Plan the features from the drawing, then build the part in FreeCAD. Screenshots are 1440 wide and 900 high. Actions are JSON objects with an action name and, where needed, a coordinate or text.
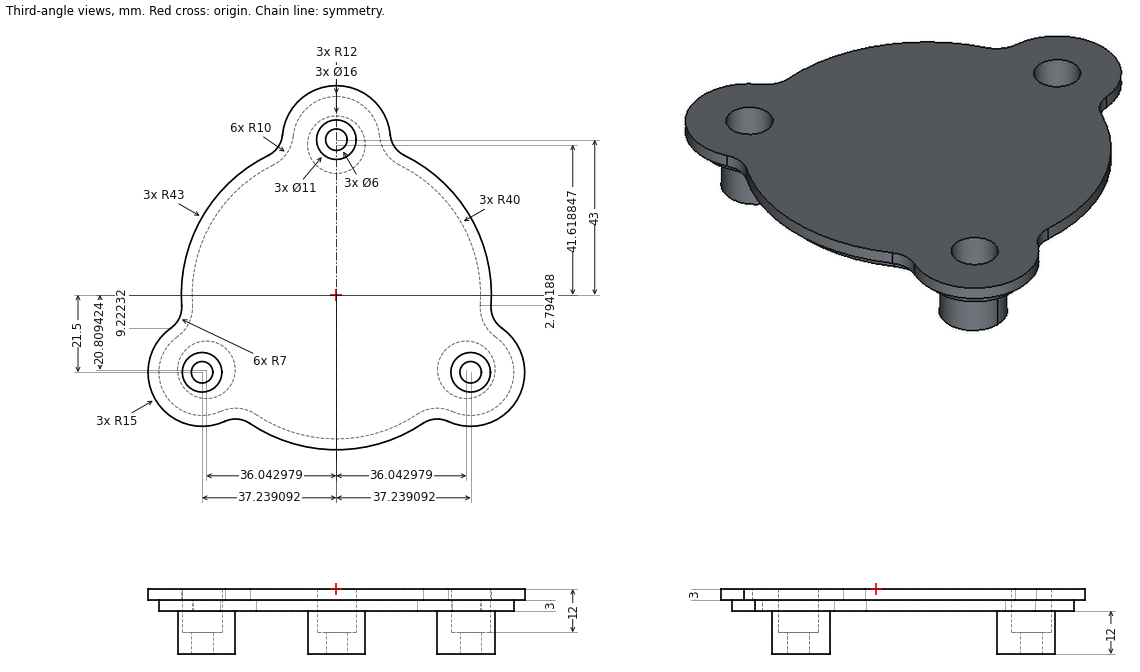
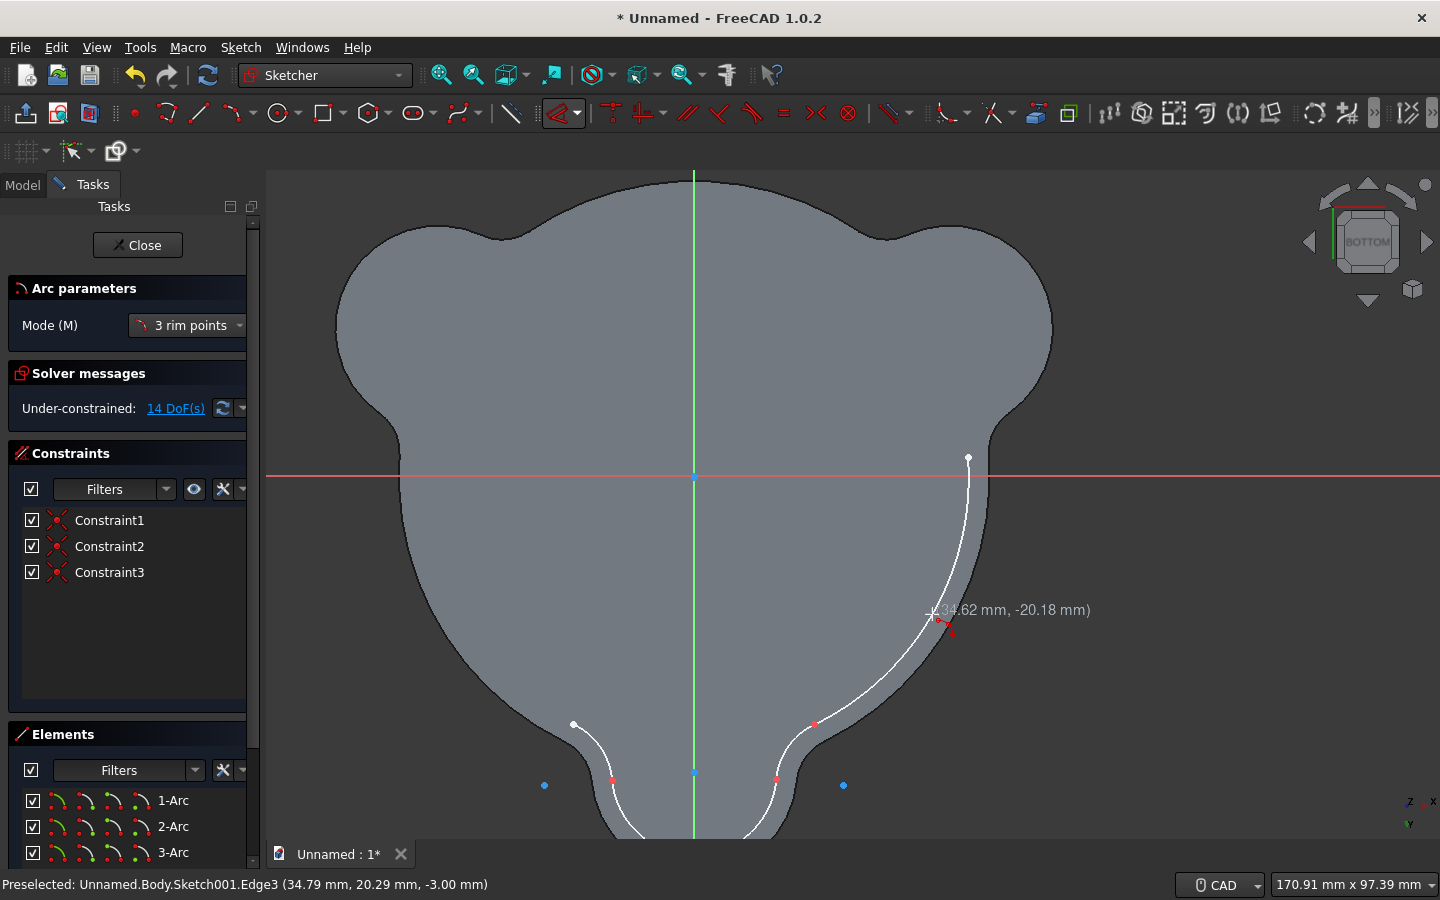
{"action": "left_click", "coordinate": [968, 458]}
{"action": "left_click", "coordinate": [997, 396]}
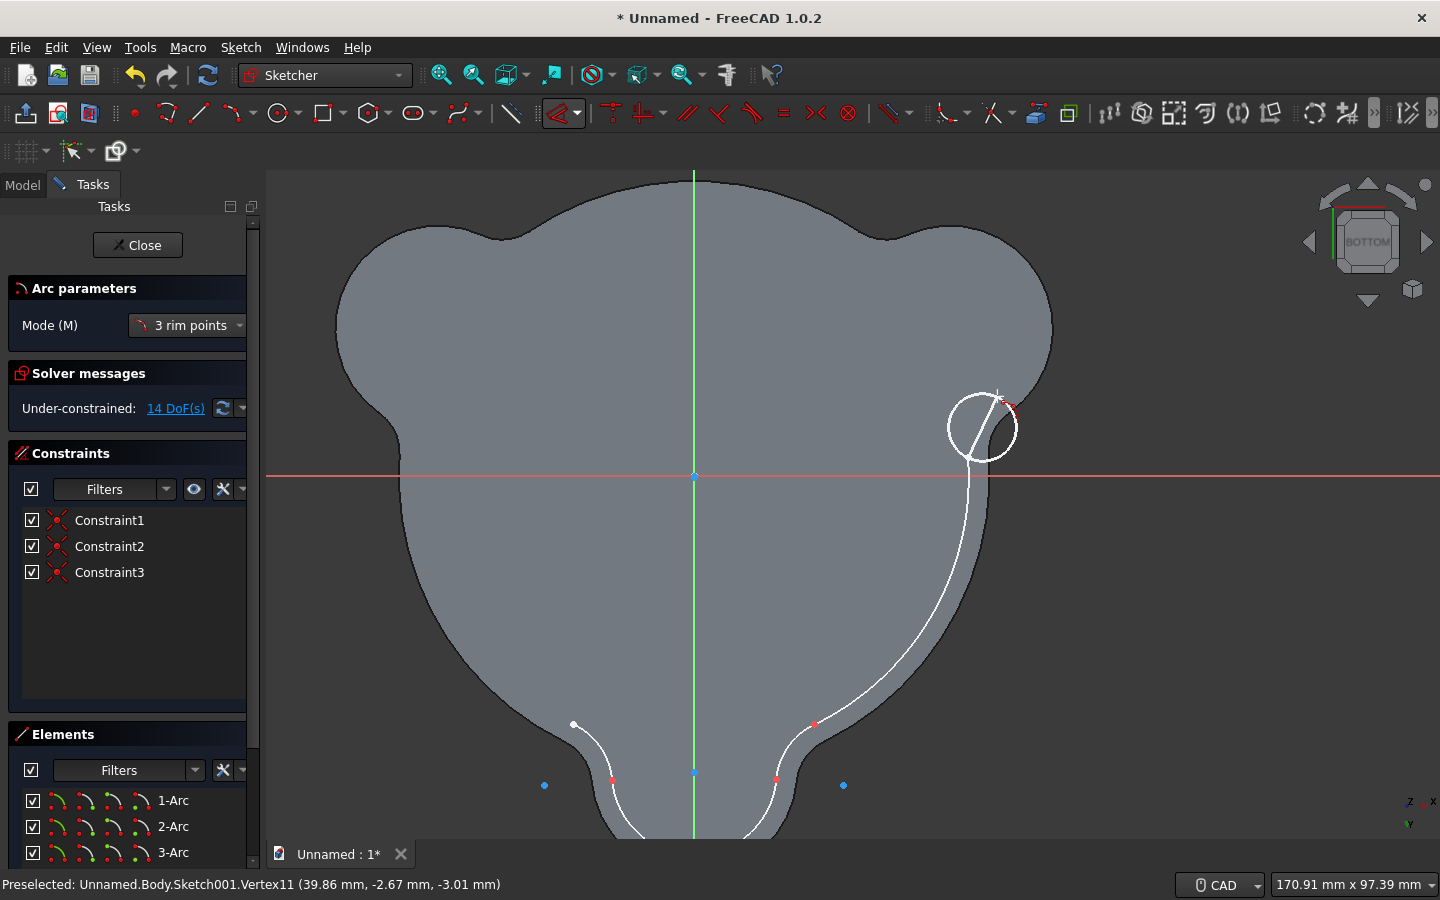
{"action": "scroll", "coordinate": [975, 423], "scroll_direction": "up", "scroll_amount": 3}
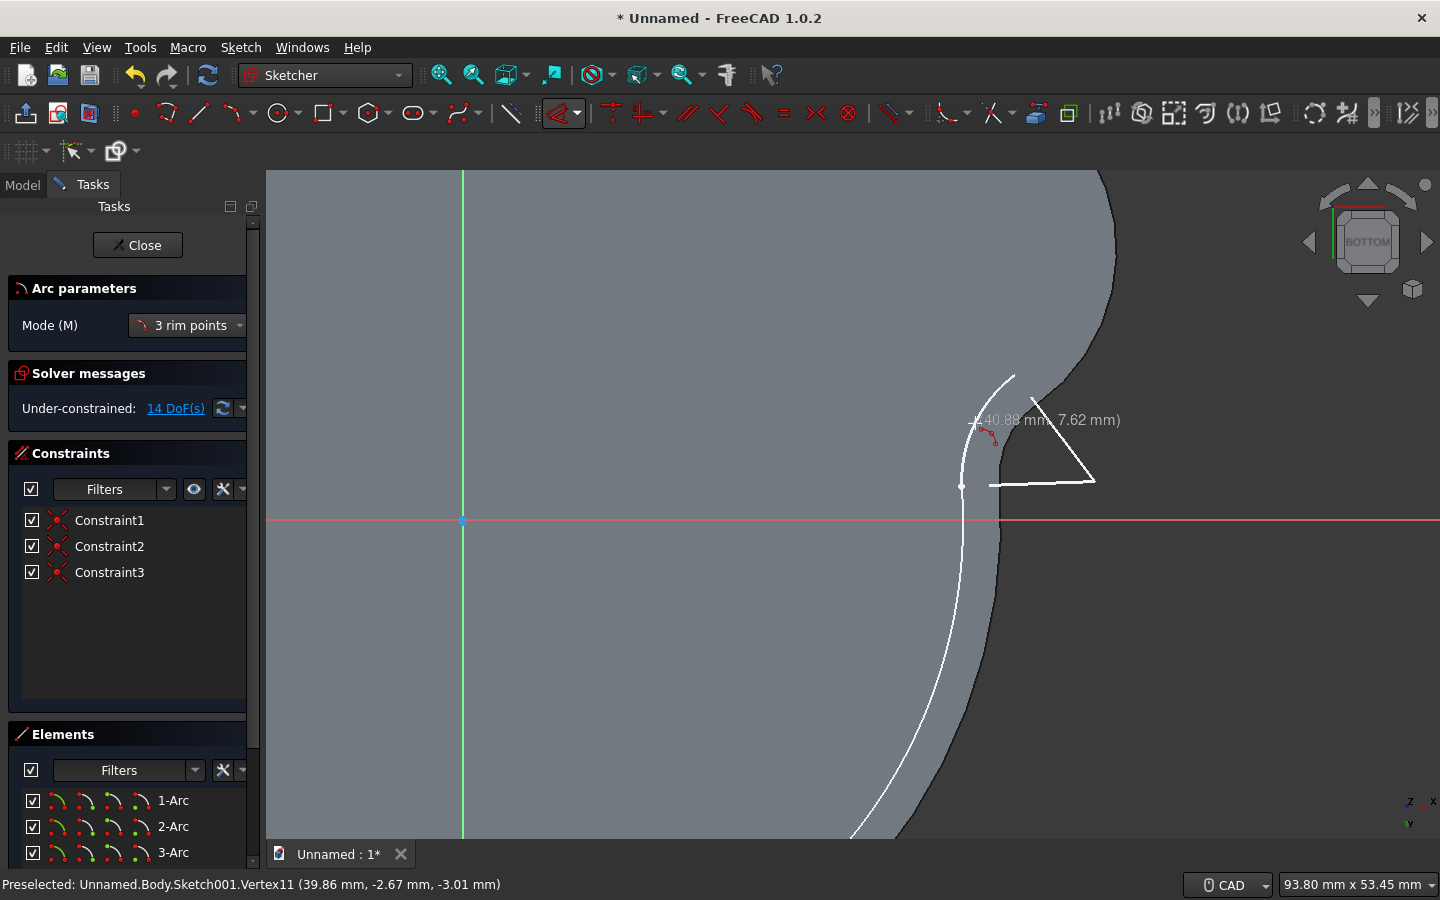
{"action": "left_click", "coordinate": [974, 422]}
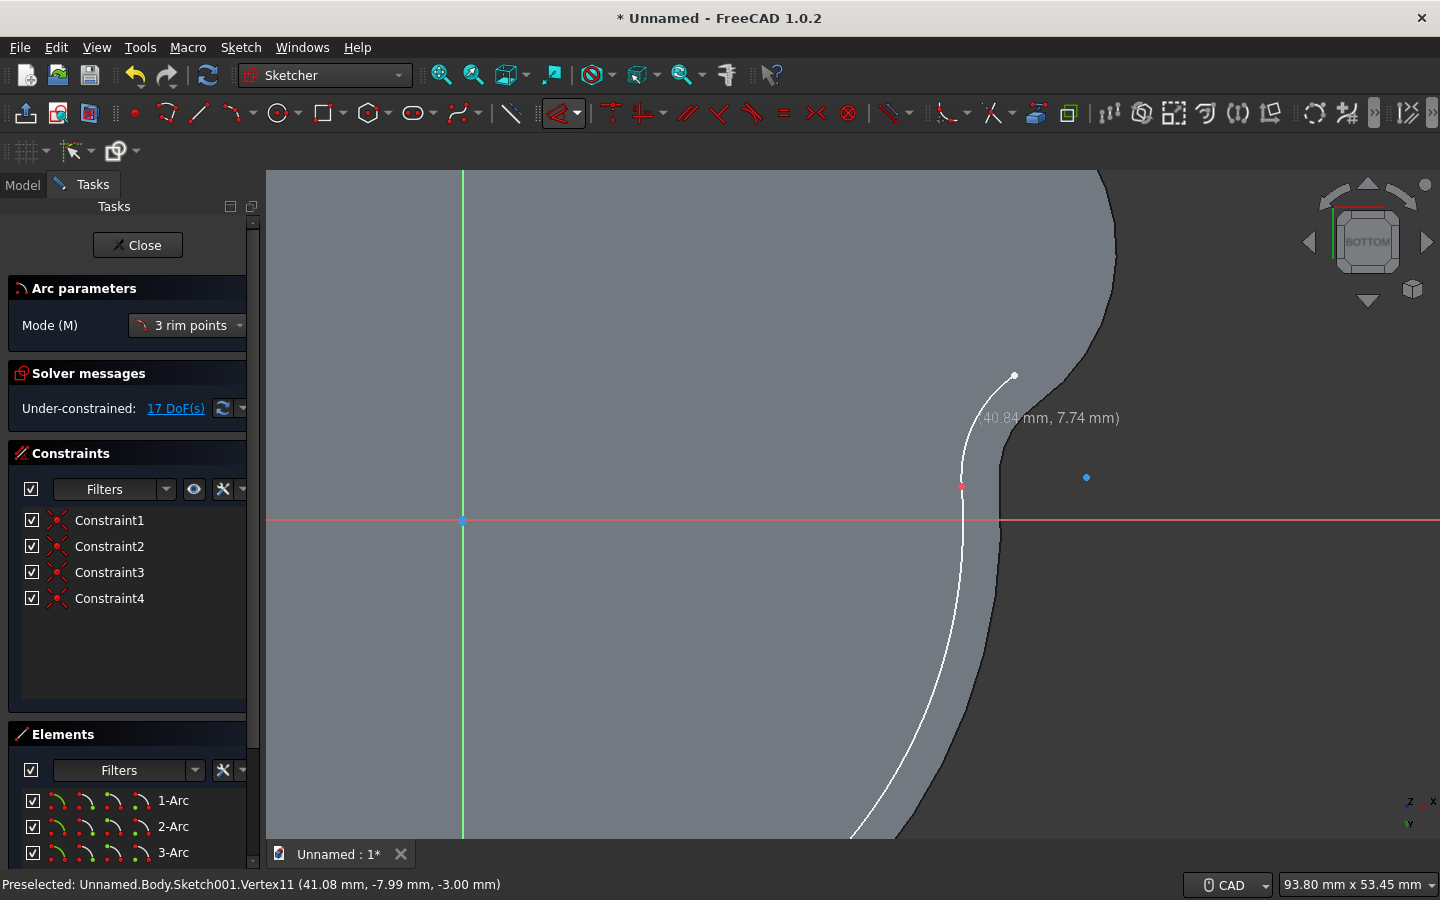
{"action": "left_click", "coordinate": [1015, 375]}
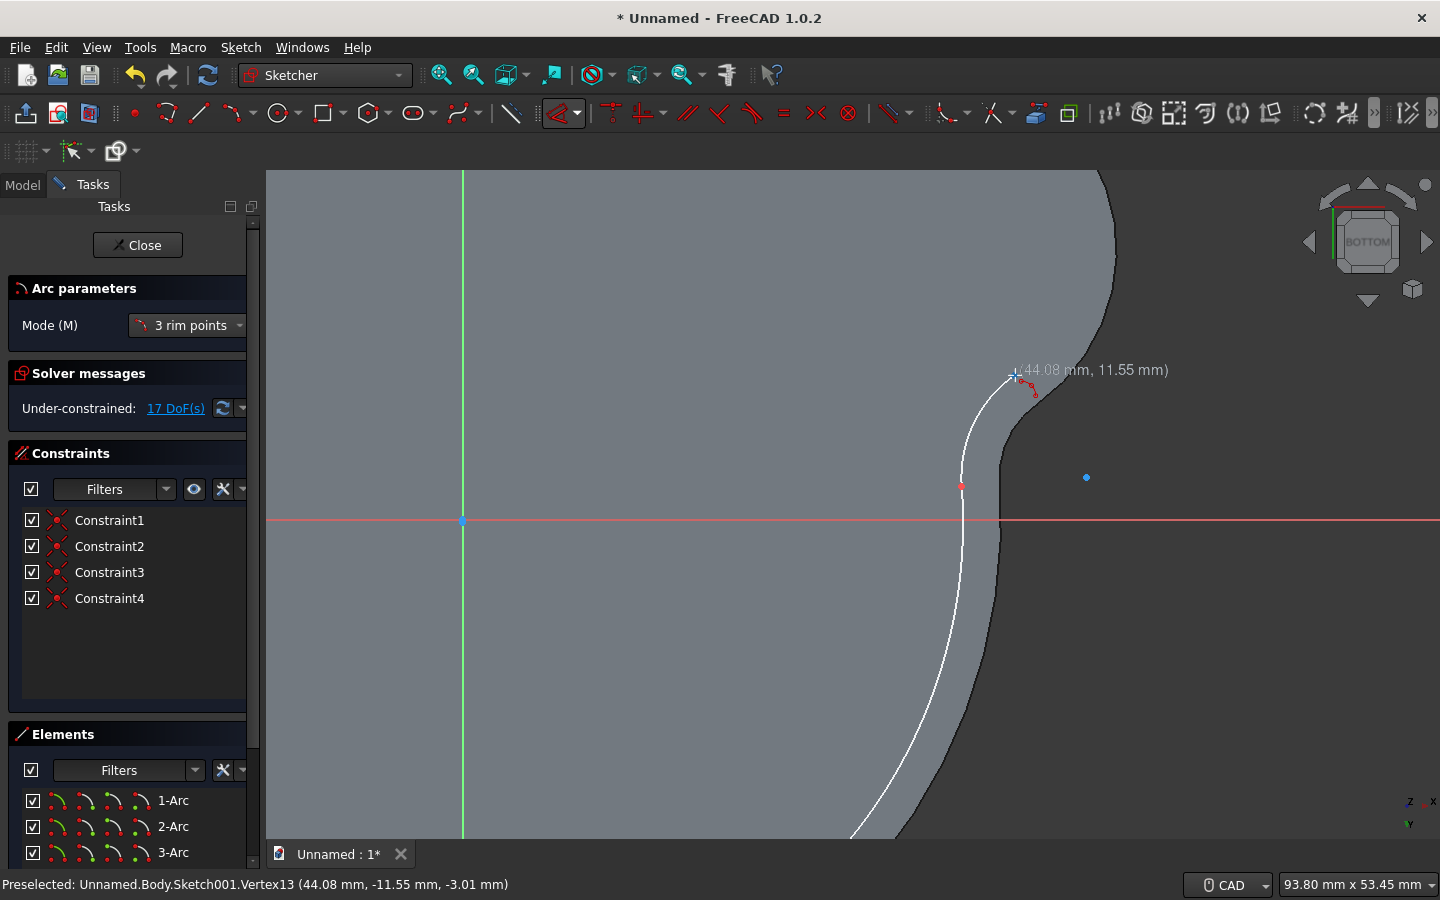
{"action": "scroll", "coordinate": [972, 441], "scroll_direction": "down", "scroll_amount": 5}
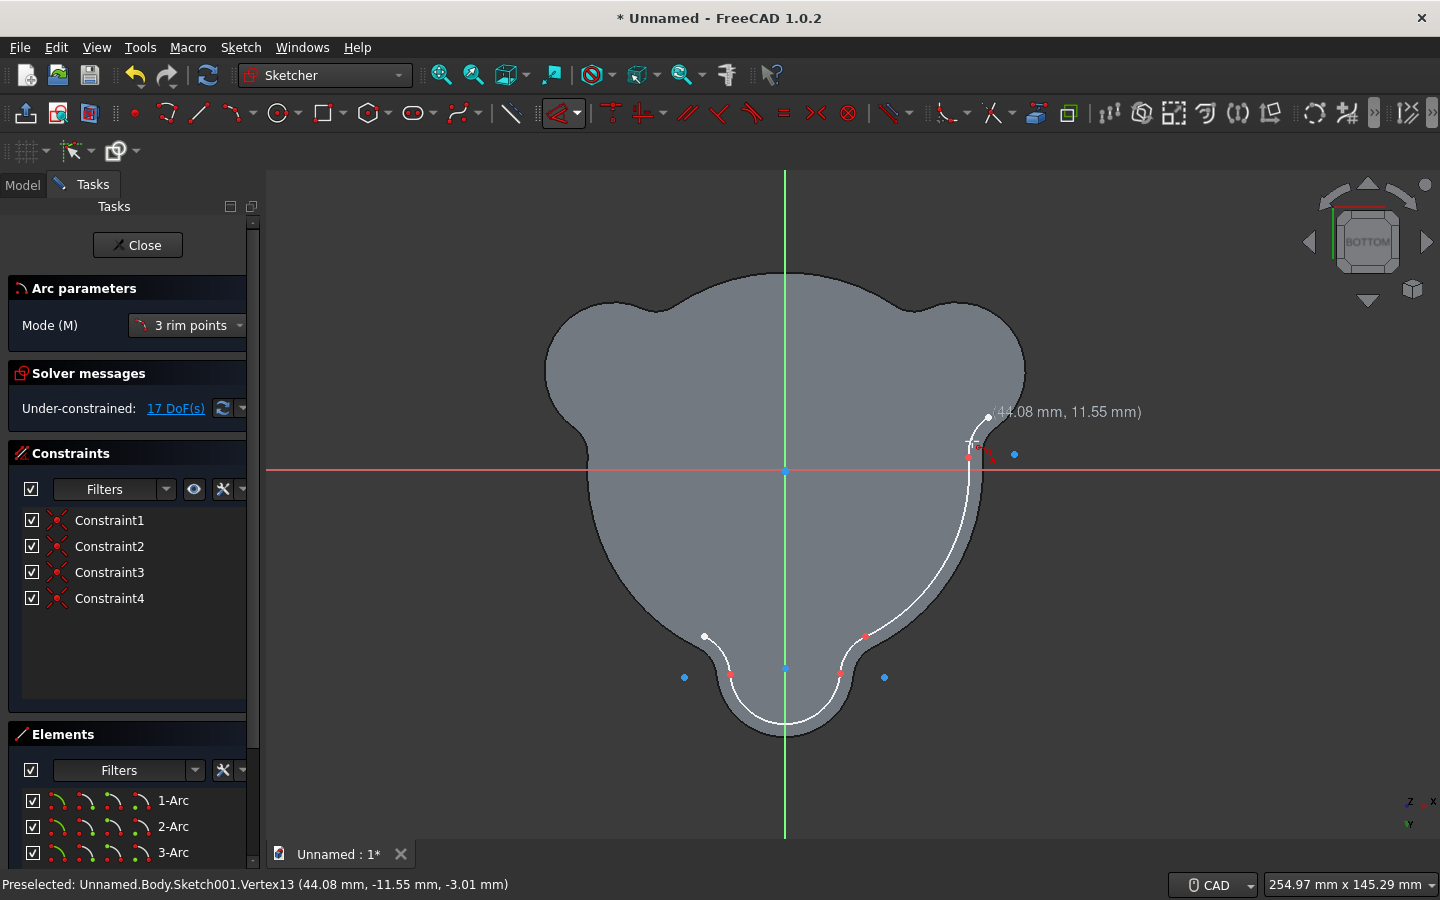
{"action": "left_click", "coordinate": [933, 321]}
{"action": "left_click", "coordinate": [1004, 344]}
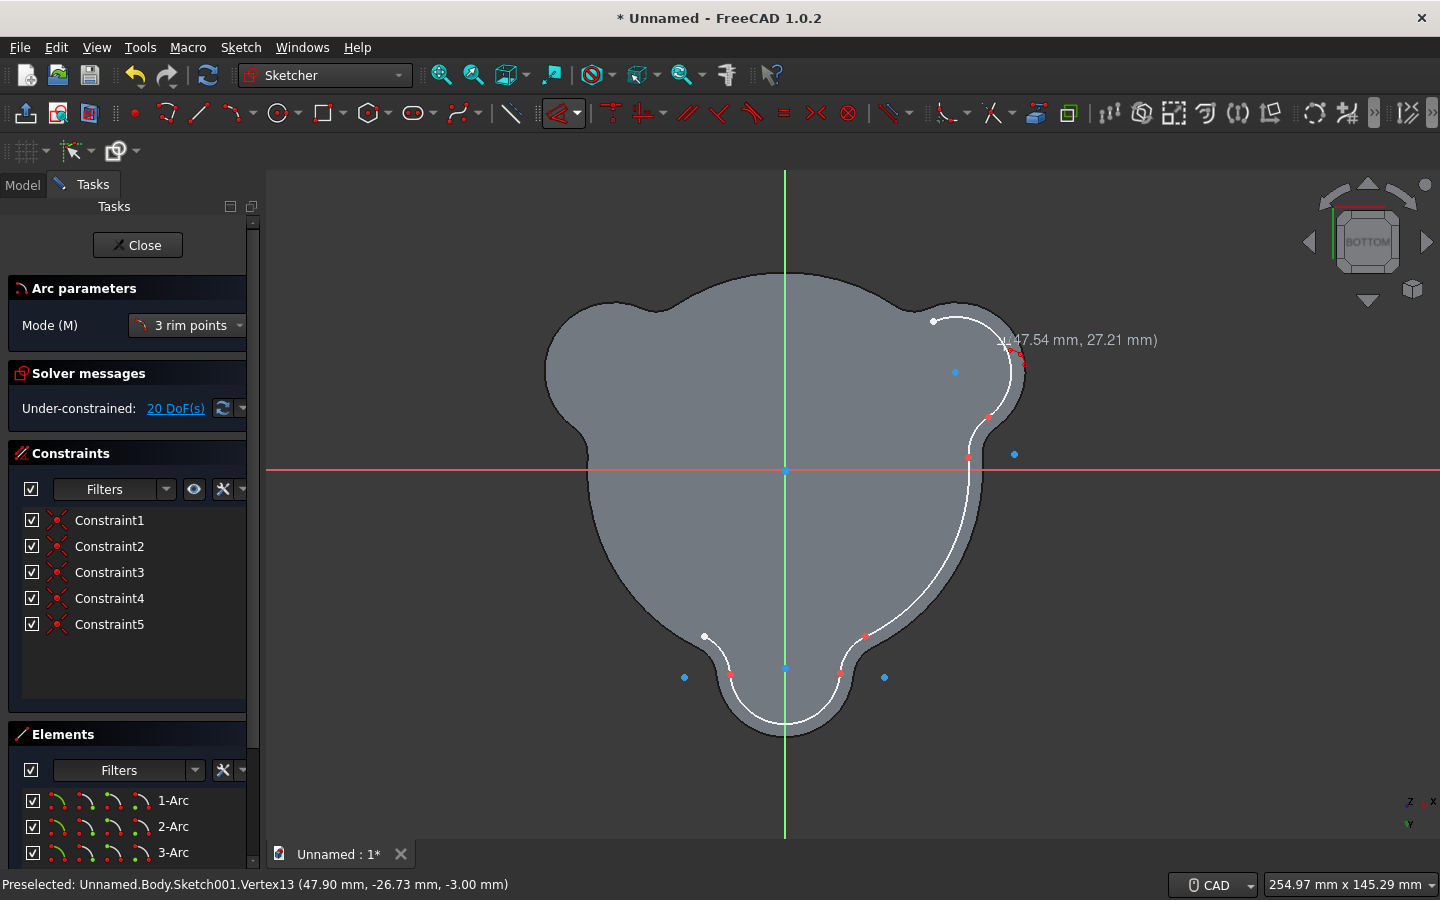
{"action": "left_click", "coordinate": [933, 322]}
{"action": "left_click", "coordinate": [888, 318]}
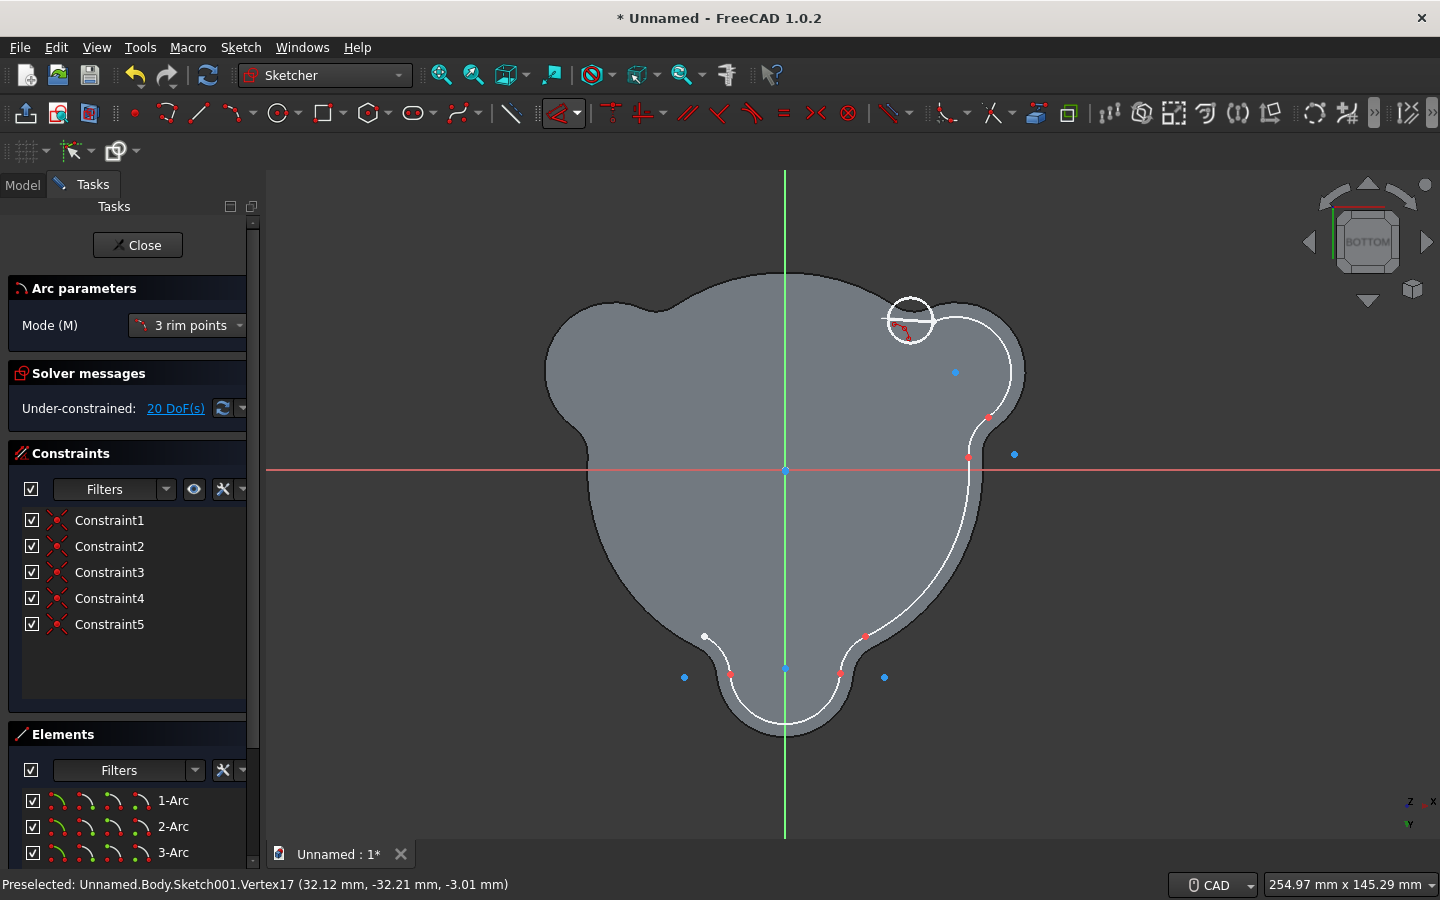
{"action": "scroll", "coordinate": [910, 325], "scroll_direction": "up", "scroll_amount": 5}